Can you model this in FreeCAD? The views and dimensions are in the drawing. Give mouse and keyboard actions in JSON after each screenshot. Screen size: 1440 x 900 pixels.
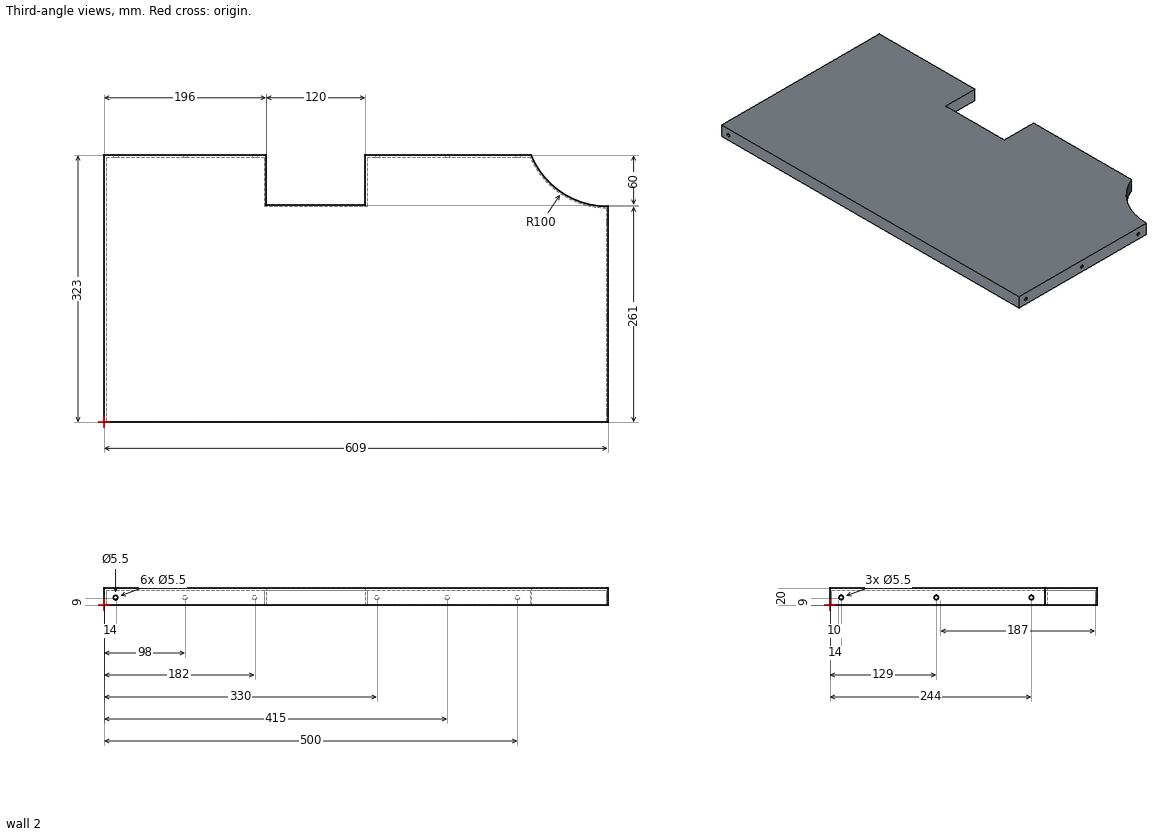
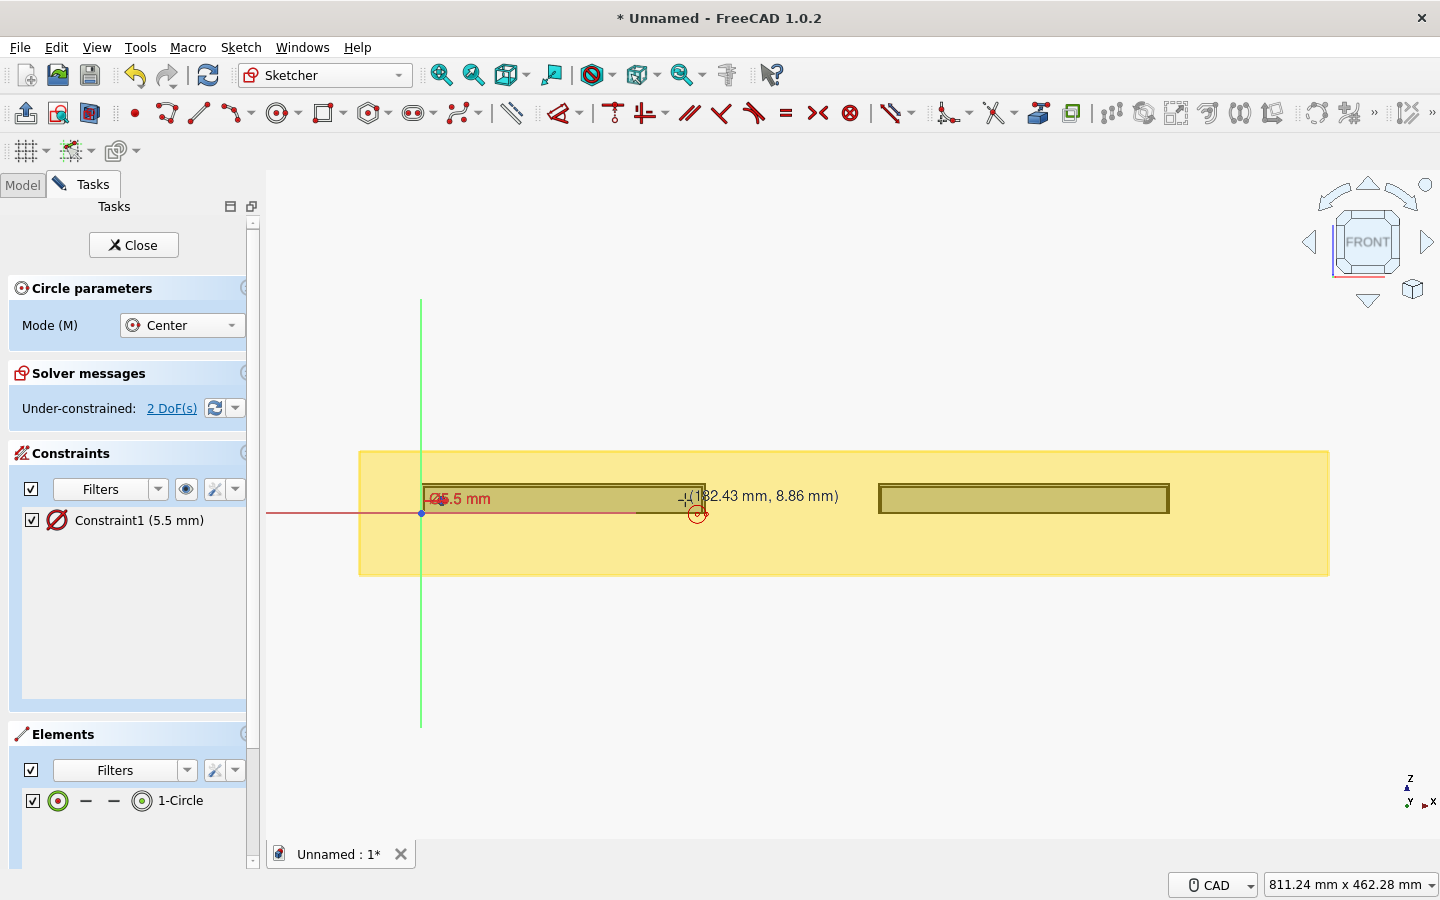
{"action": "left_click", "coordinate": [685, 500]}
{"action": "mouse_move", "coordinate": [687, 498]}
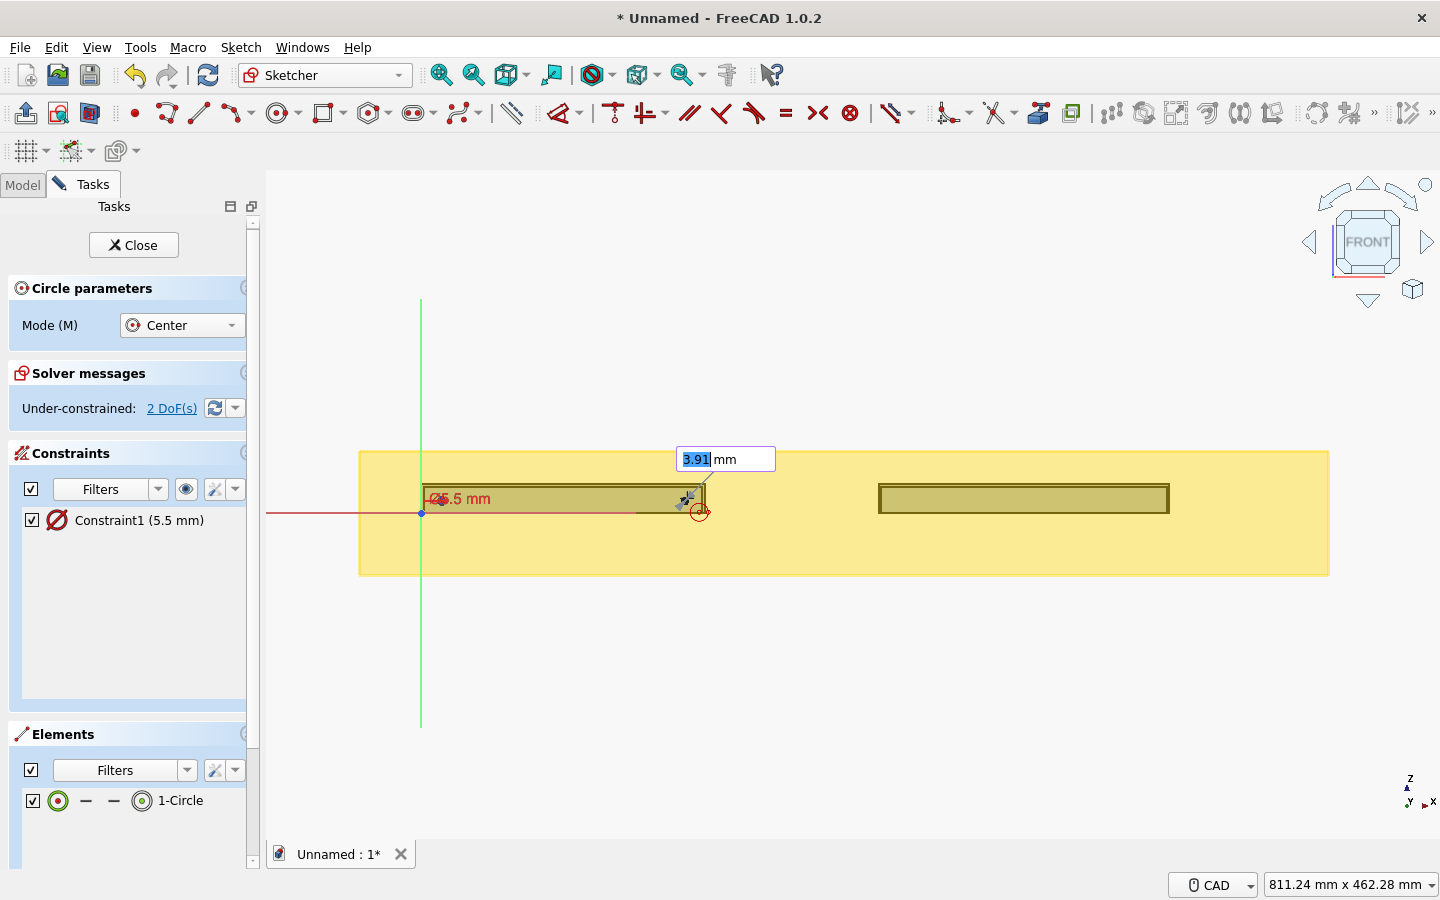
{"action": "type", "text": "5.5"}
{"action": "key", "text": "Return"}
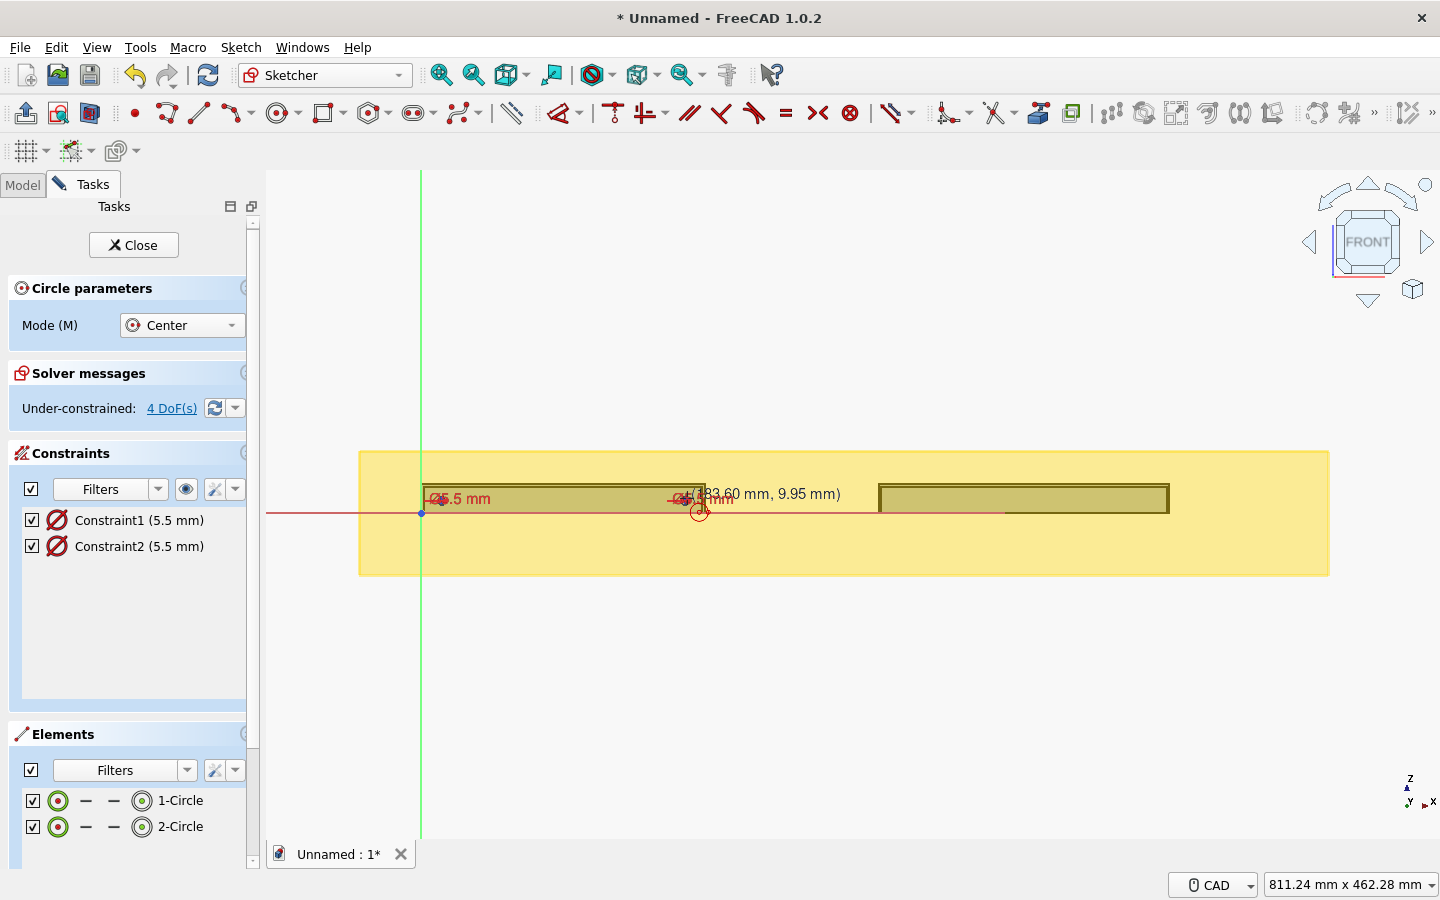
{"action": "scroll", "coordinate": [563, 500], "scroll_direction": "up", "scroll_amount": 9}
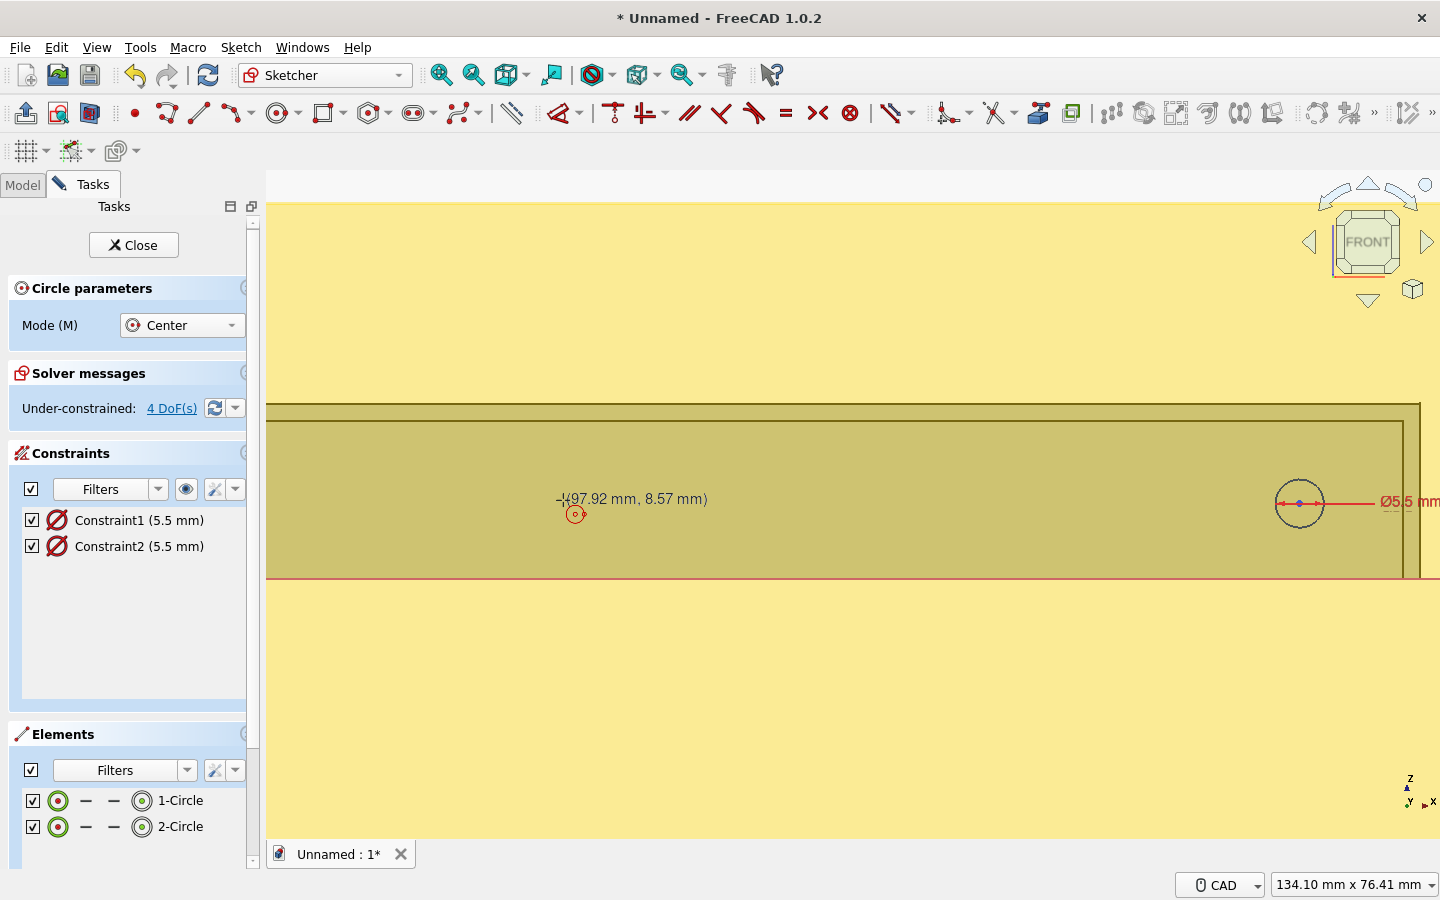
{"action": "scroll", "coordinate": [563, 500], "scroll_direction": "down", "scroll_amount": 9}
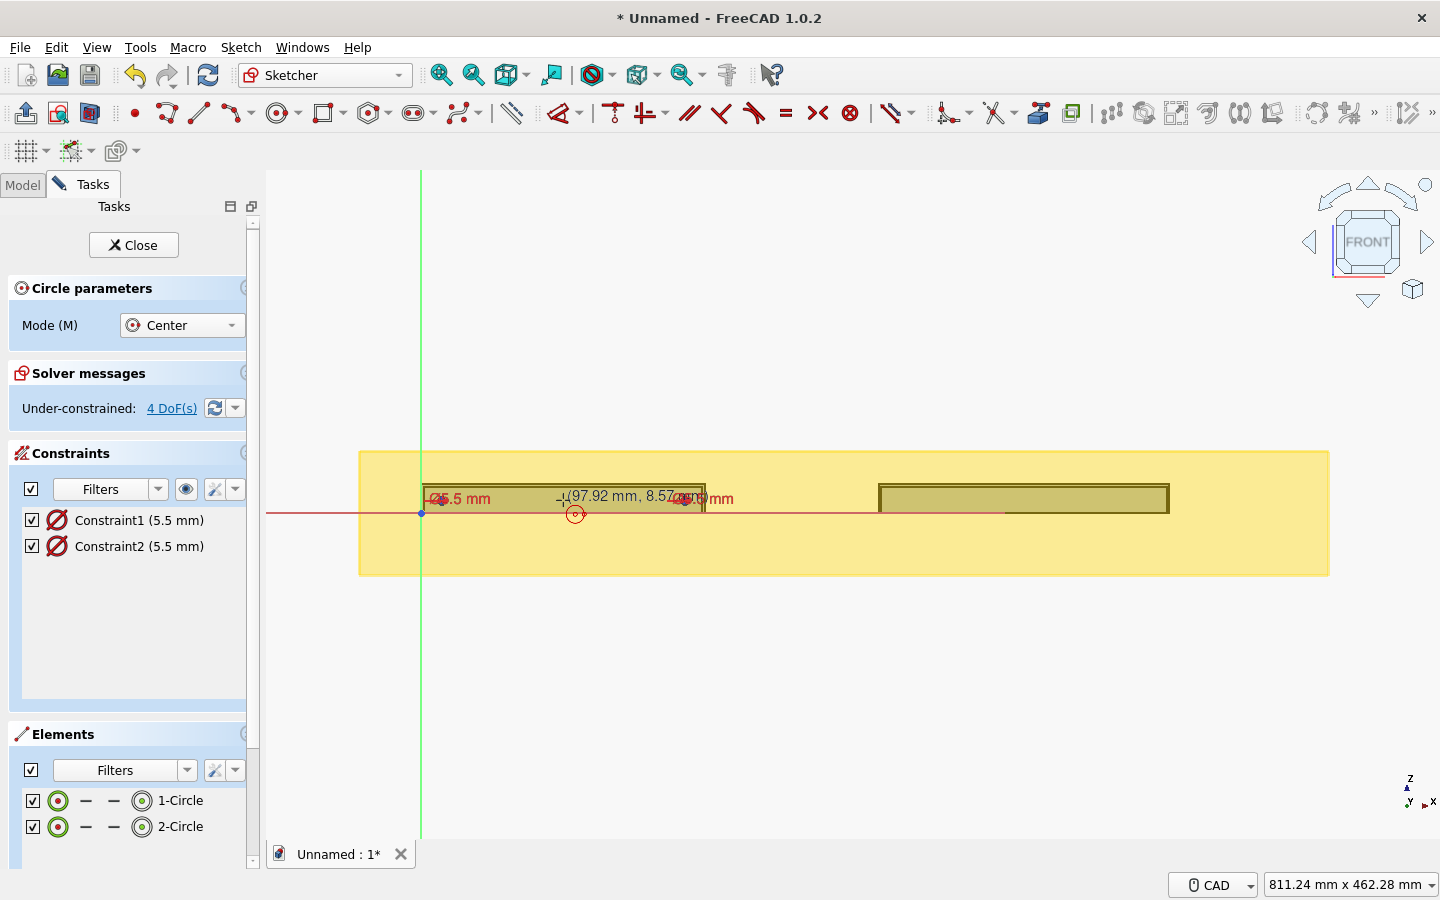
{"action": "left_click", "coordinate": [563, 500]}
{"action": "mouse_move", "coordinate": [566, 498]}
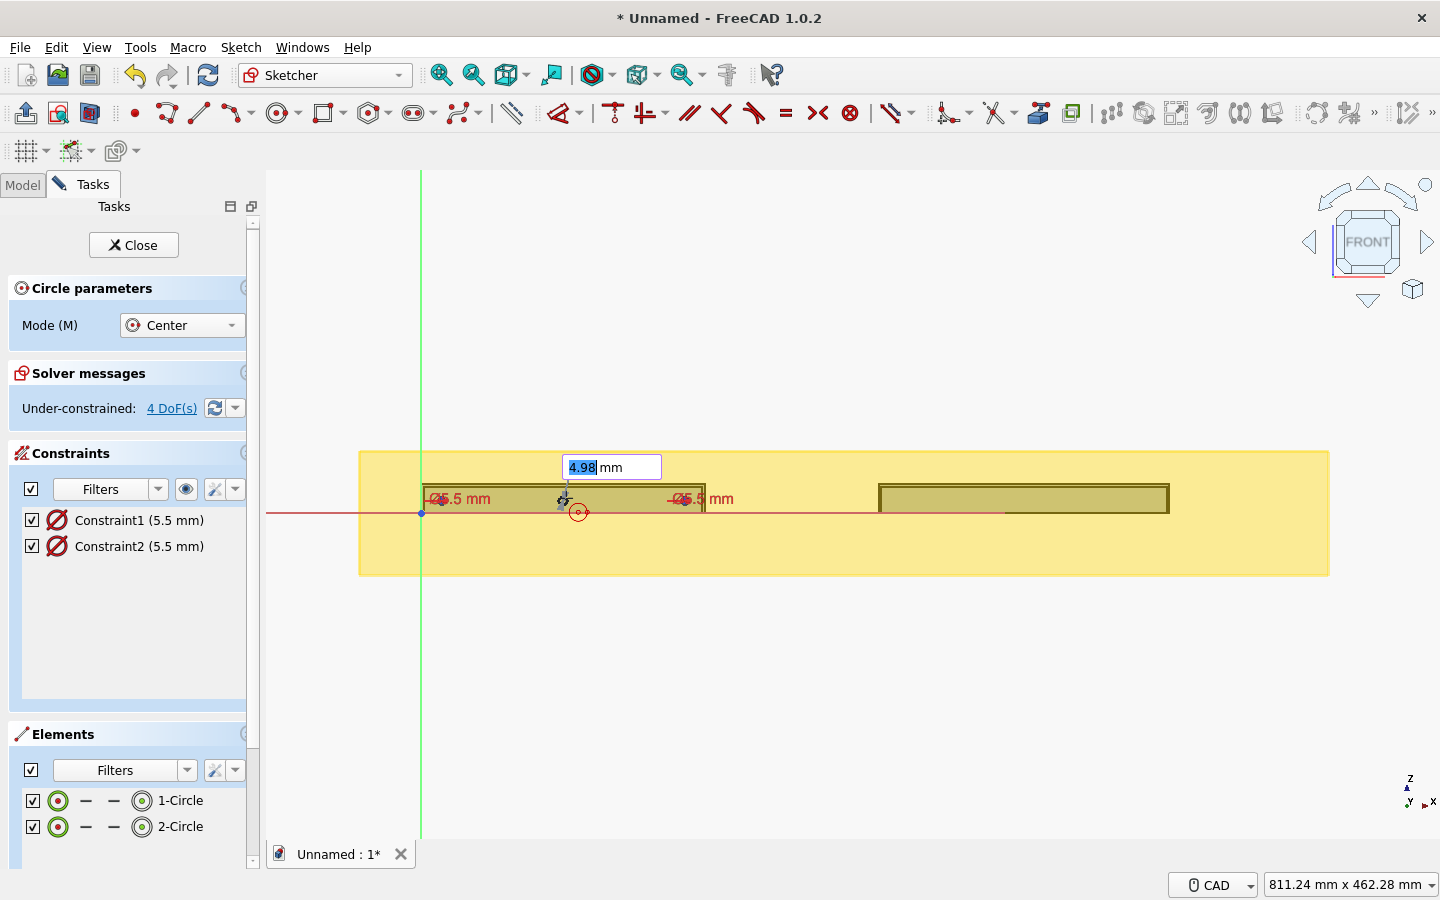
{"action": "type", "text": "5.5"}
{"action": "key", "text": "Return"}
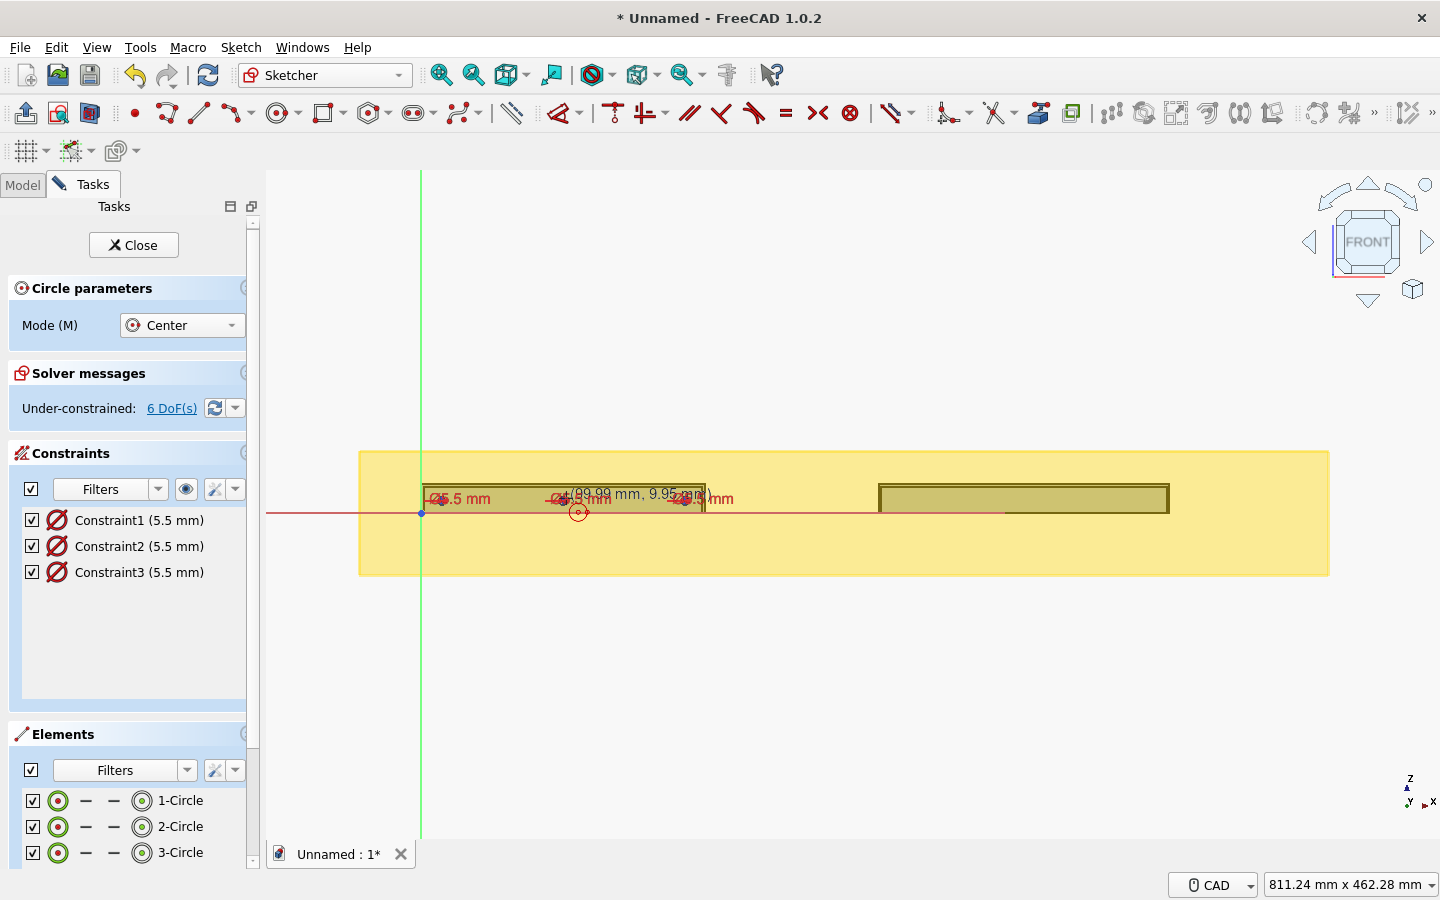
{"action": "scroll", "coordinate": [899, 500], "scroll_direction": "up", "scroll_amount": 9}